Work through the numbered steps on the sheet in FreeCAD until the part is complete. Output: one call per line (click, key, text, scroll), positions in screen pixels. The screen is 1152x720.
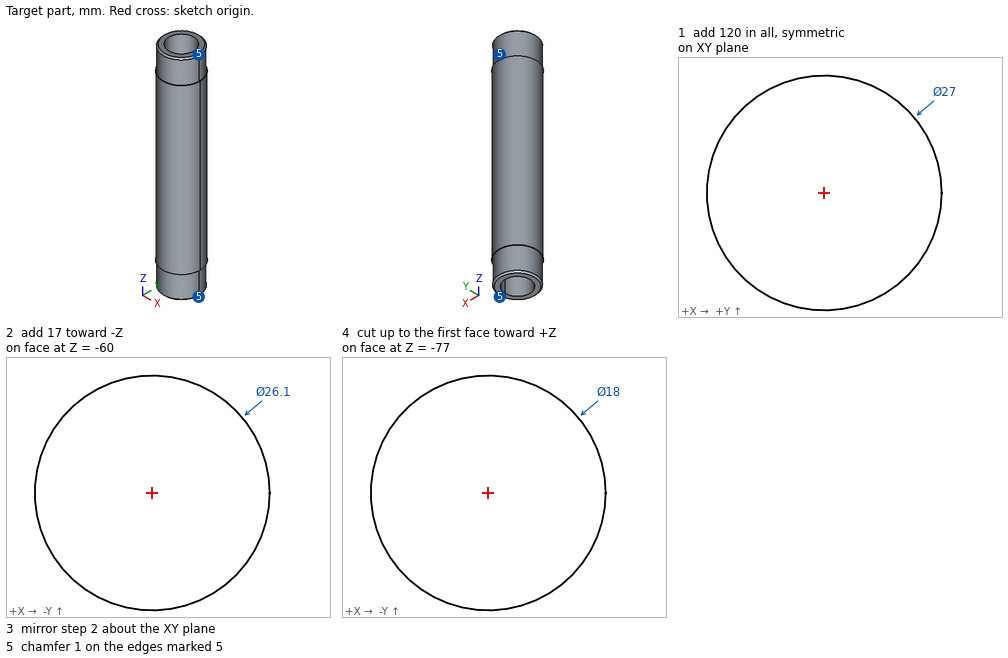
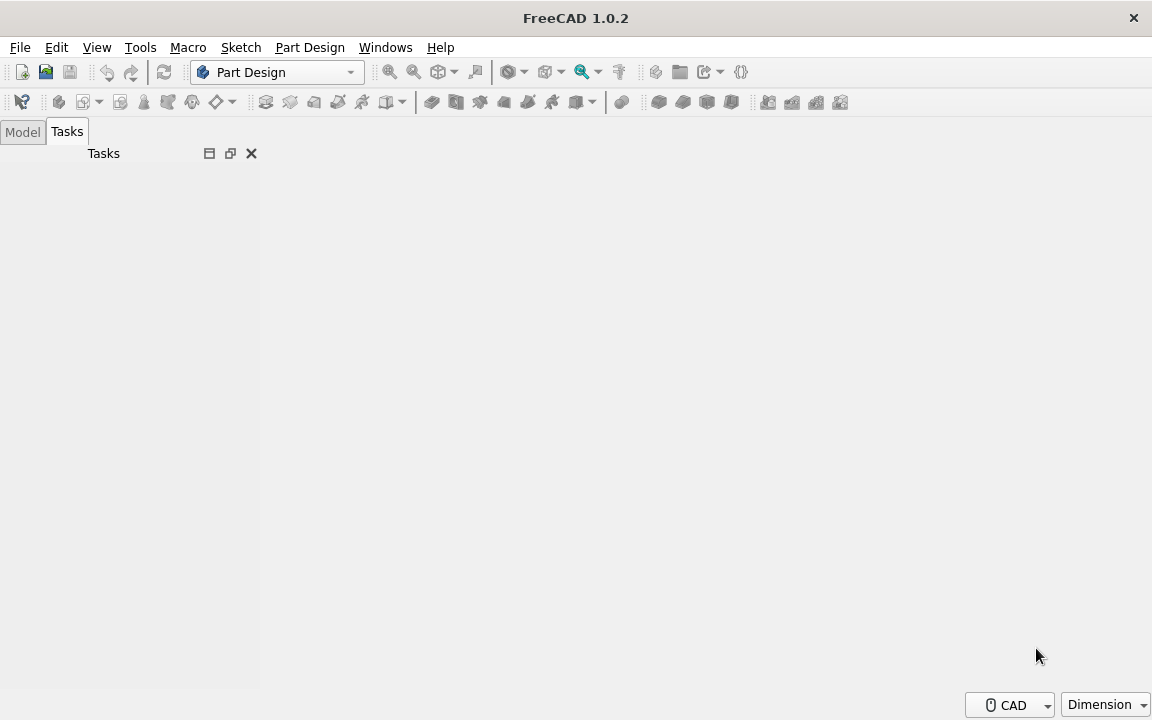
key(ctrl+n)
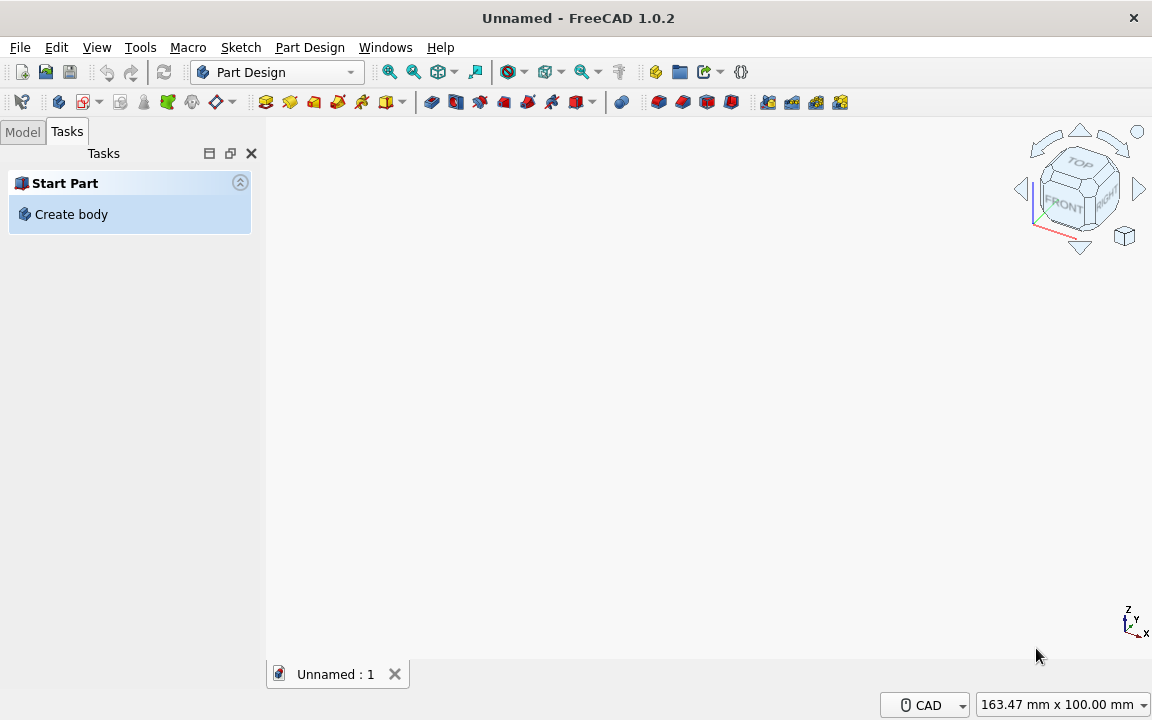
click(84, 102)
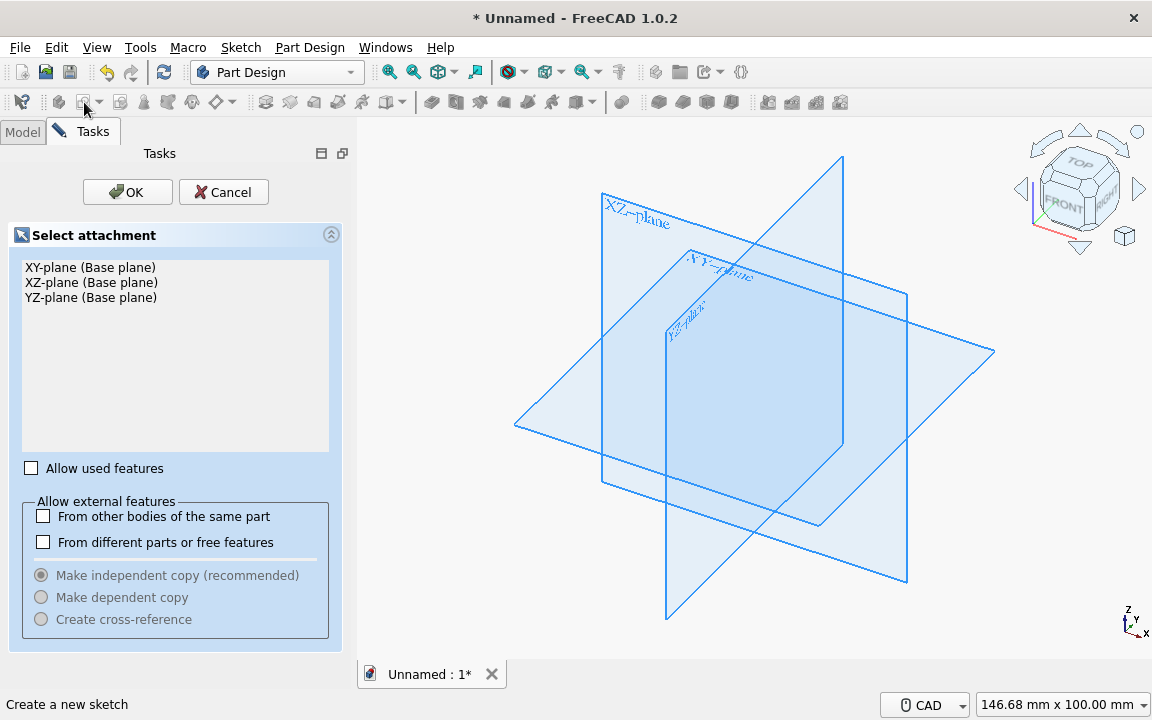
click(82, 268)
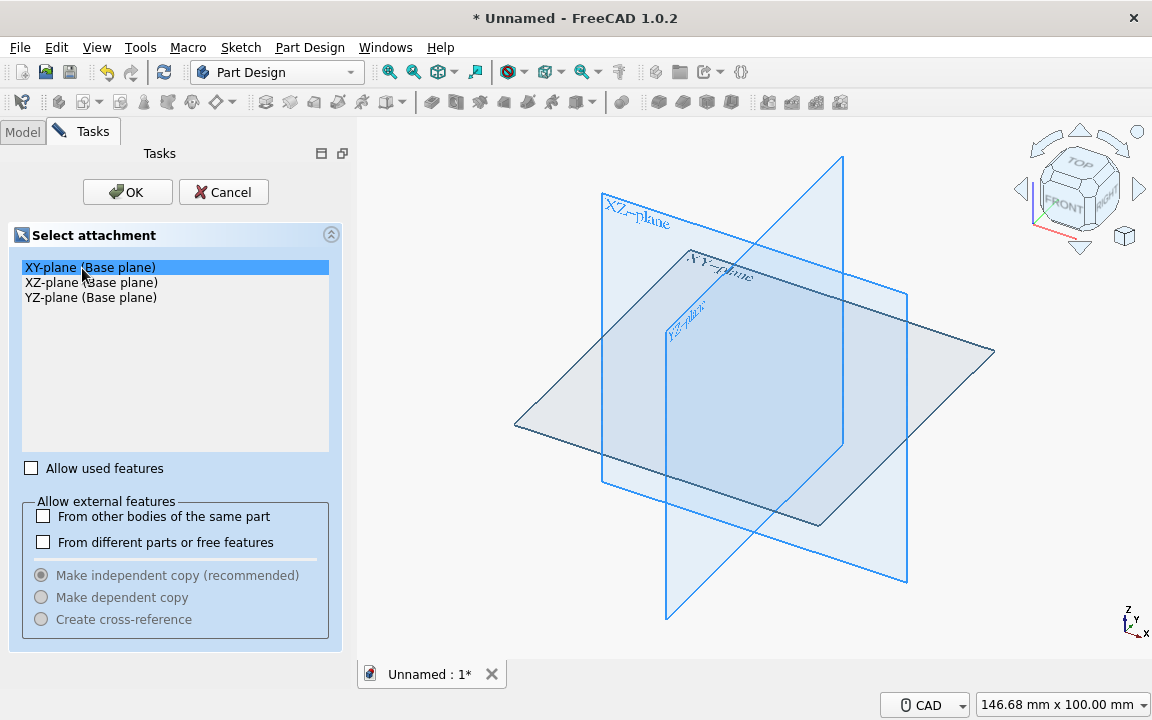
click(128, 192)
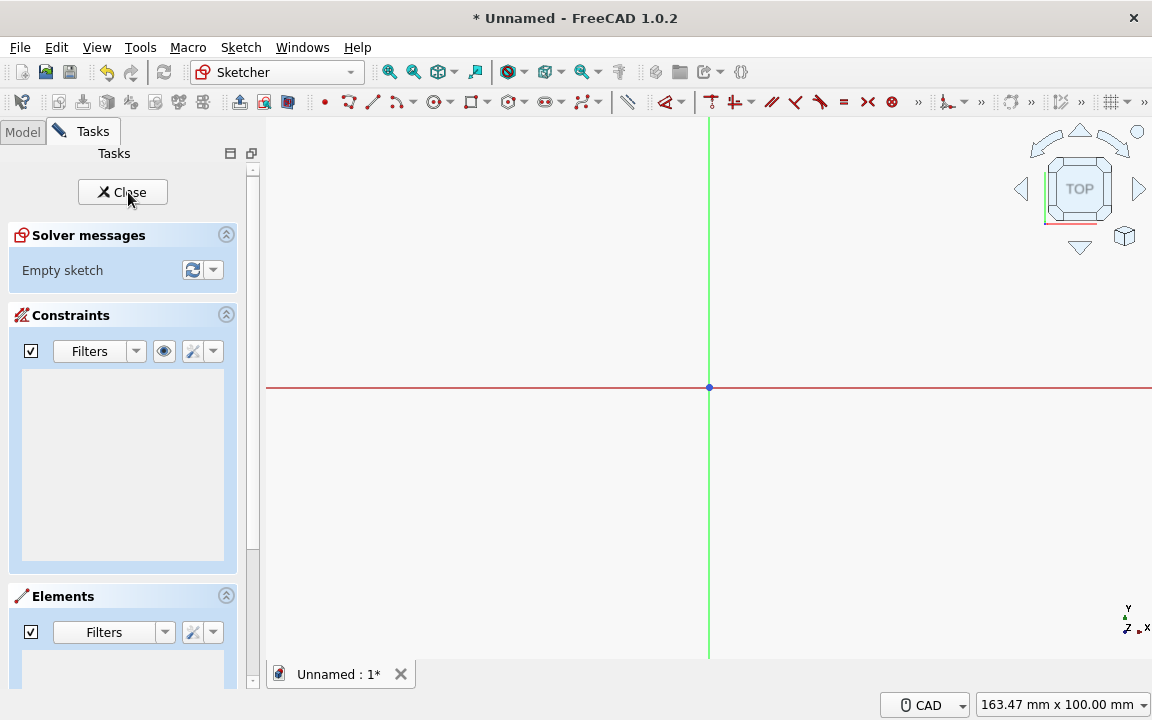
scroll(765, 388, up, 4)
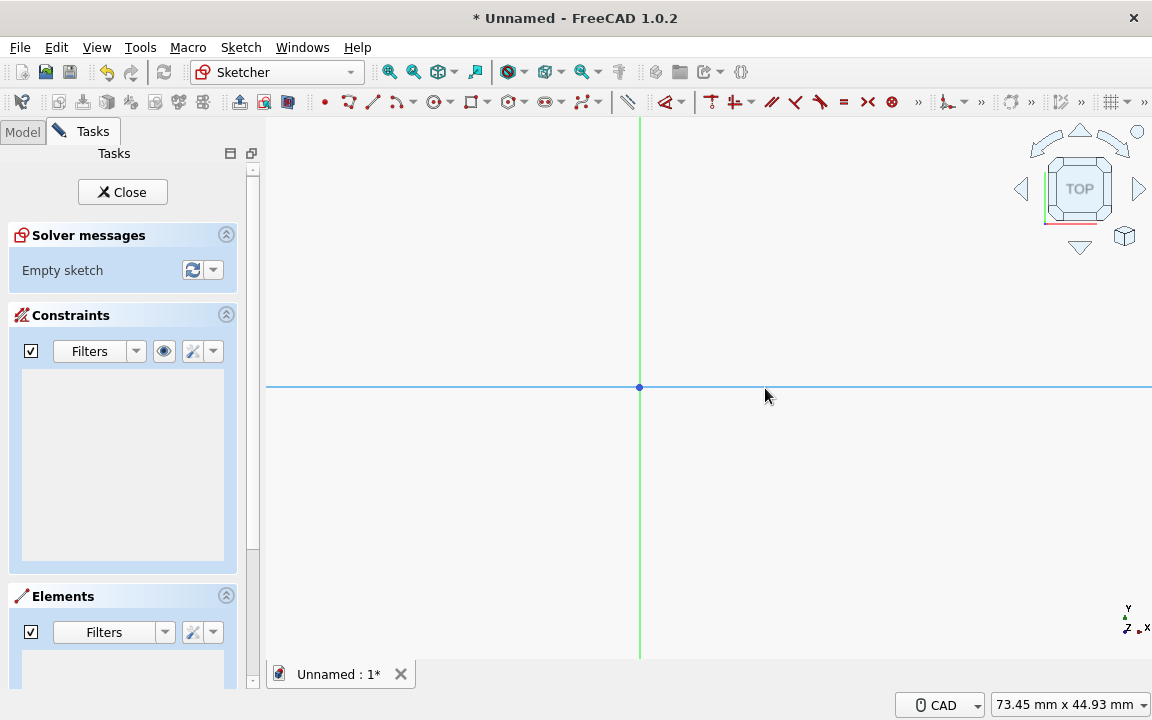
click(434, 102)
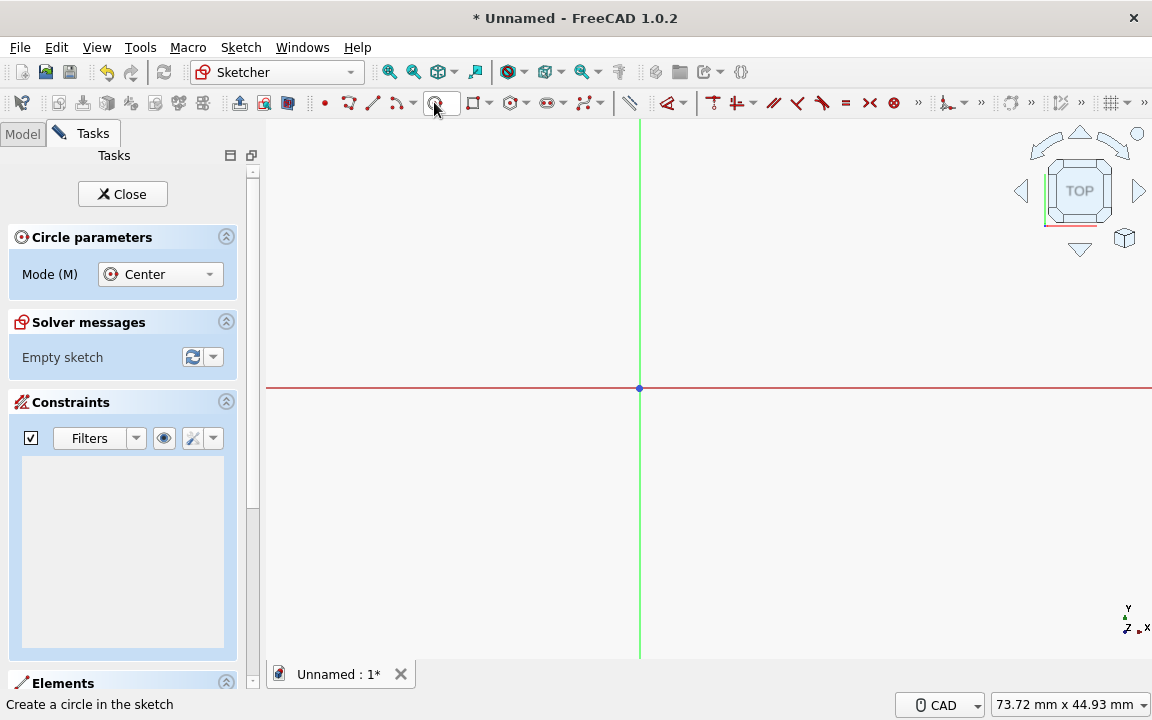
click(640, 388)
move(755, 274)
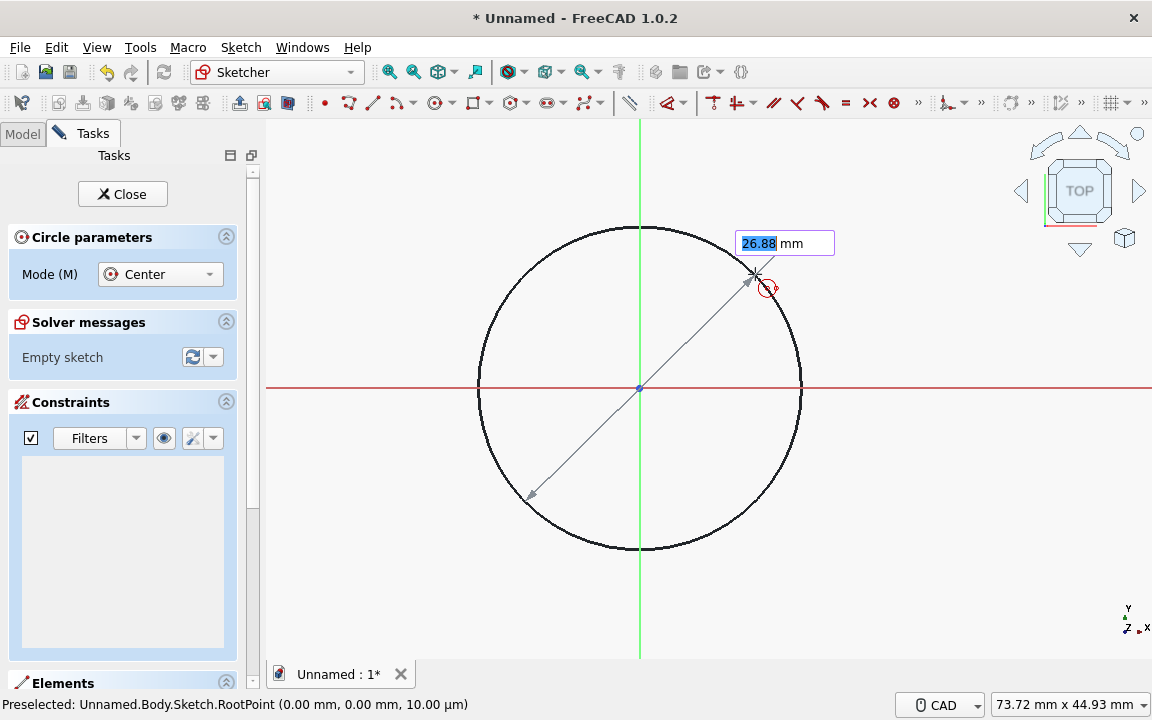
text(27)
key(Return)
key(Escape)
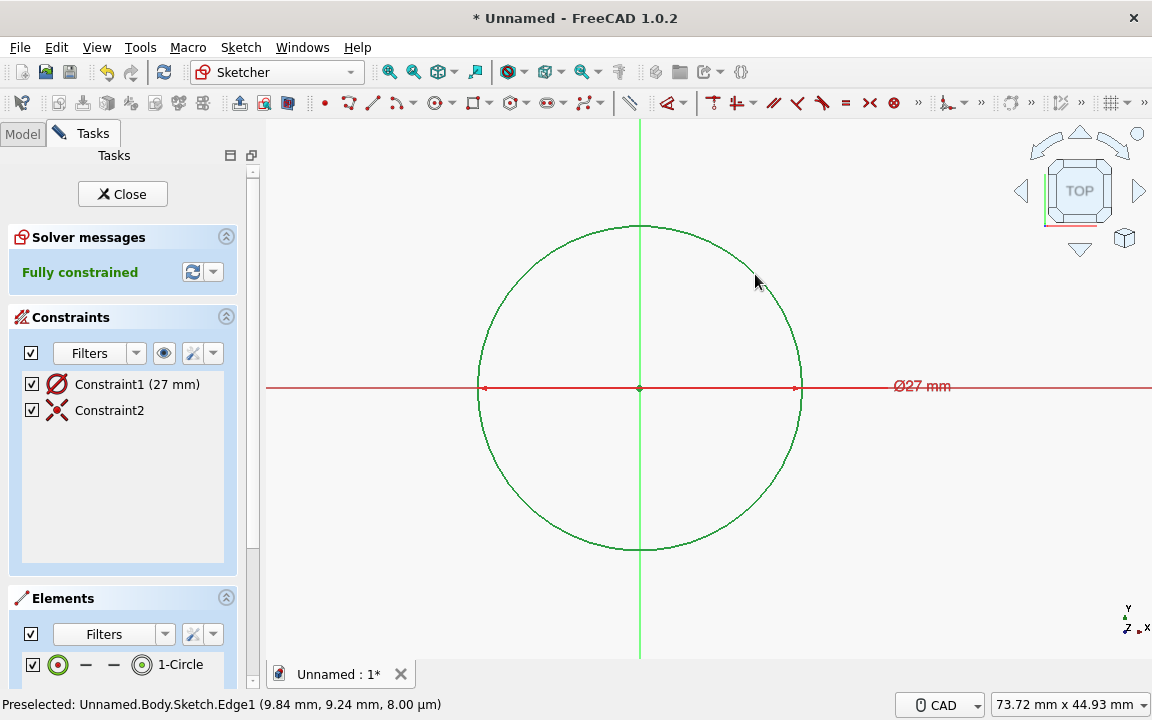
click(123, 194)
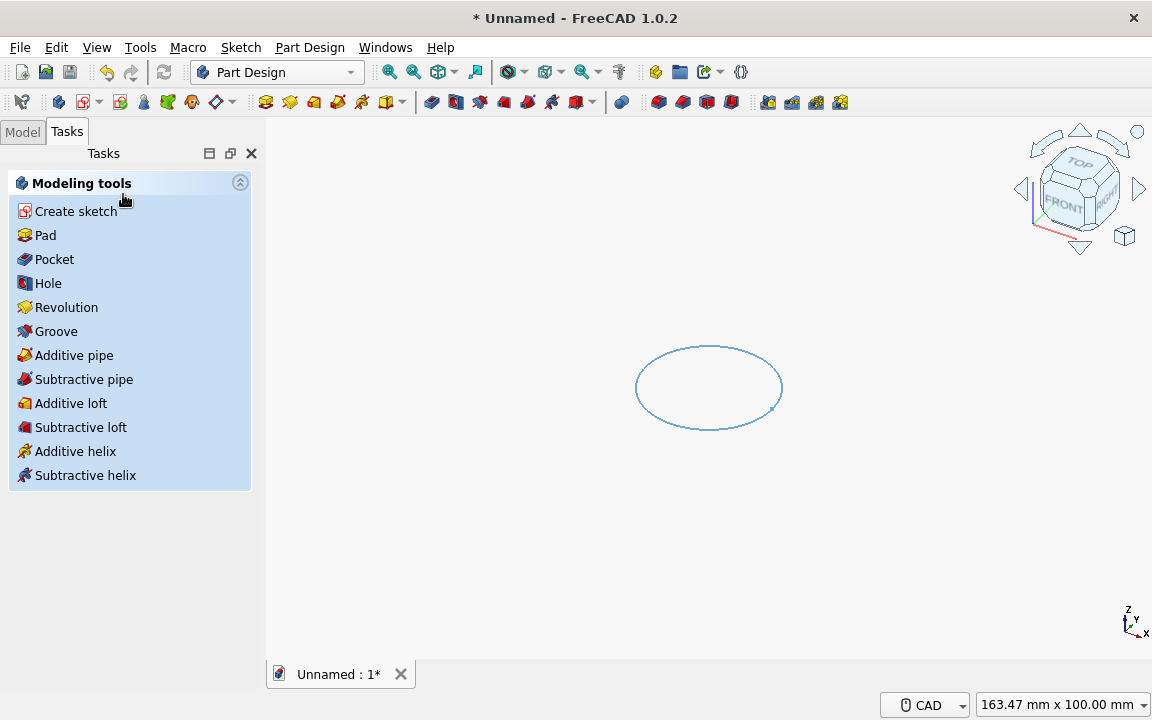
click(266, 102)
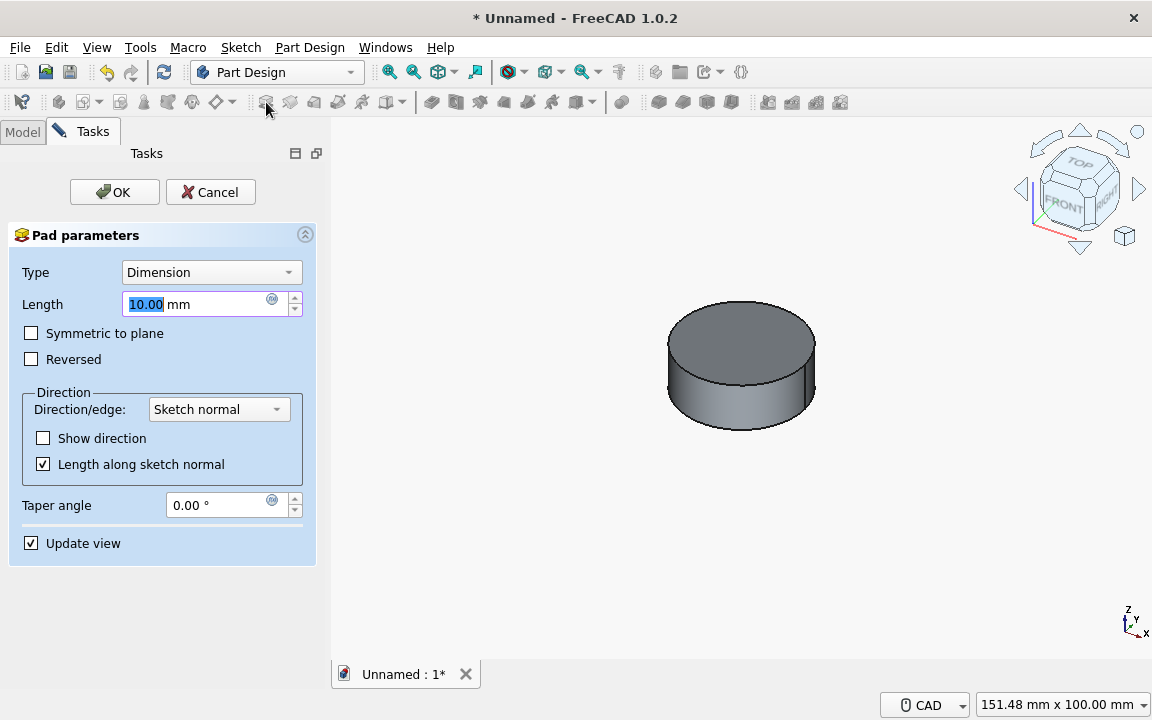
text(120)
key(Tab)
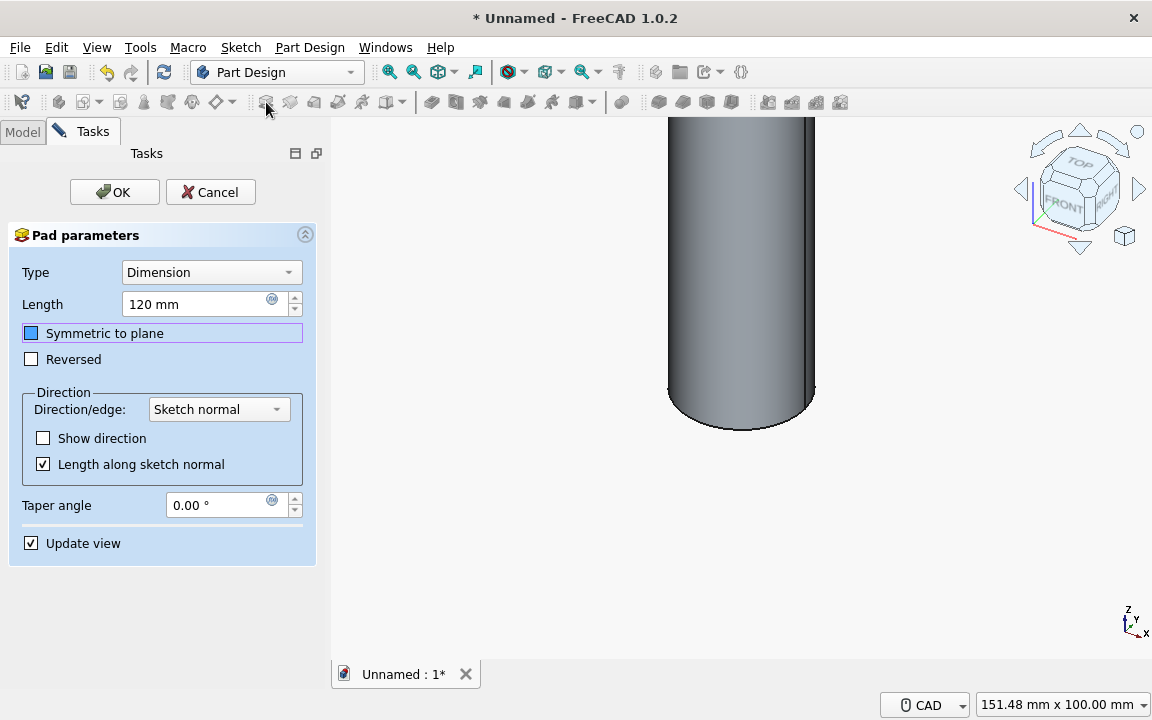
click(30, 333)